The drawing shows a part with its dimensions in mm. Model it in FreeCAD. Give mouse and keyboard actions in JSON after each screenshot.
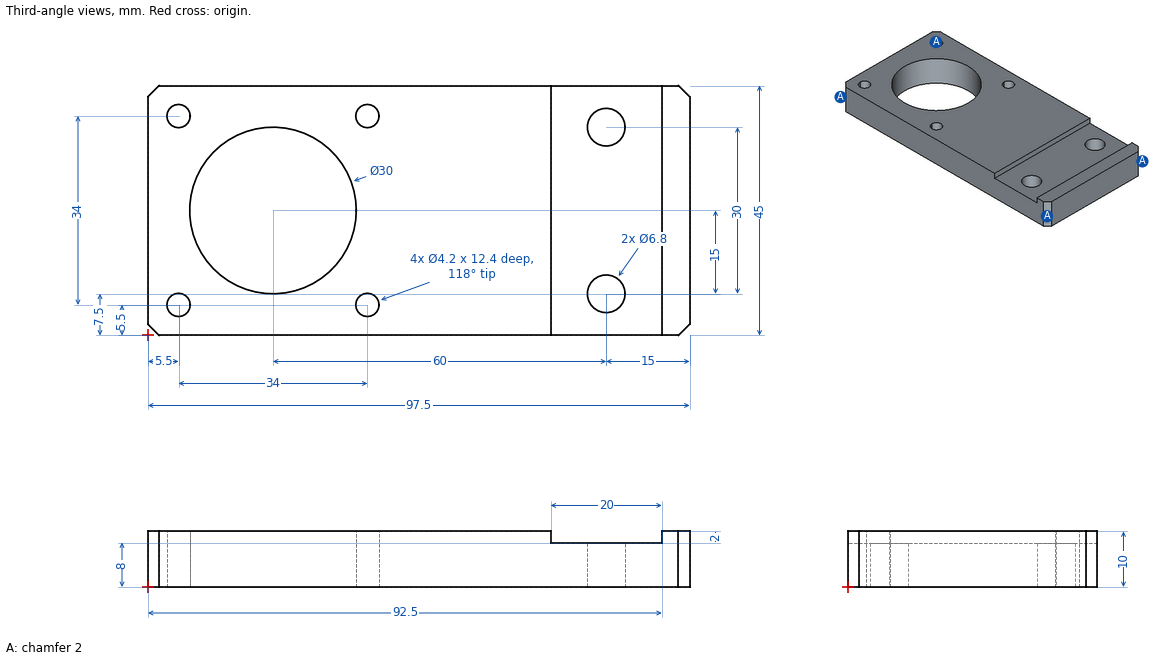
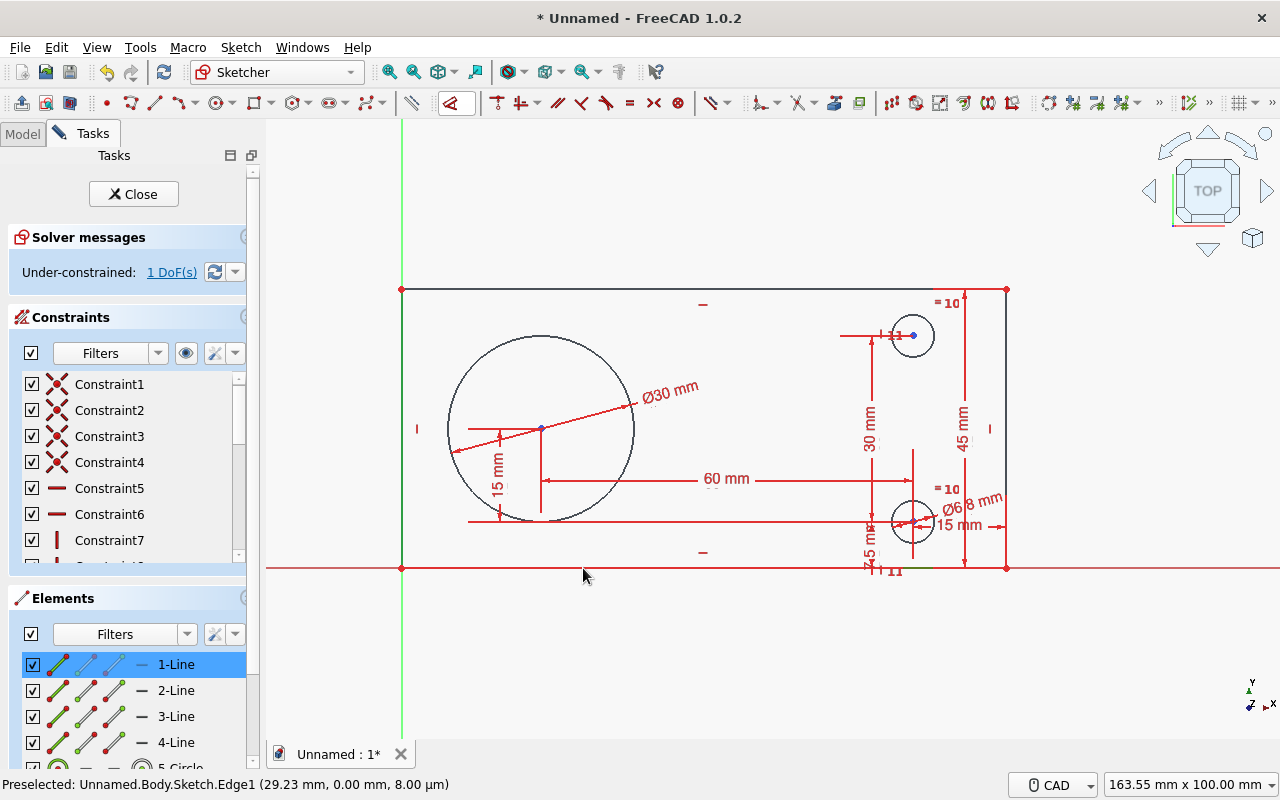
{"action": "key", "text": "l"}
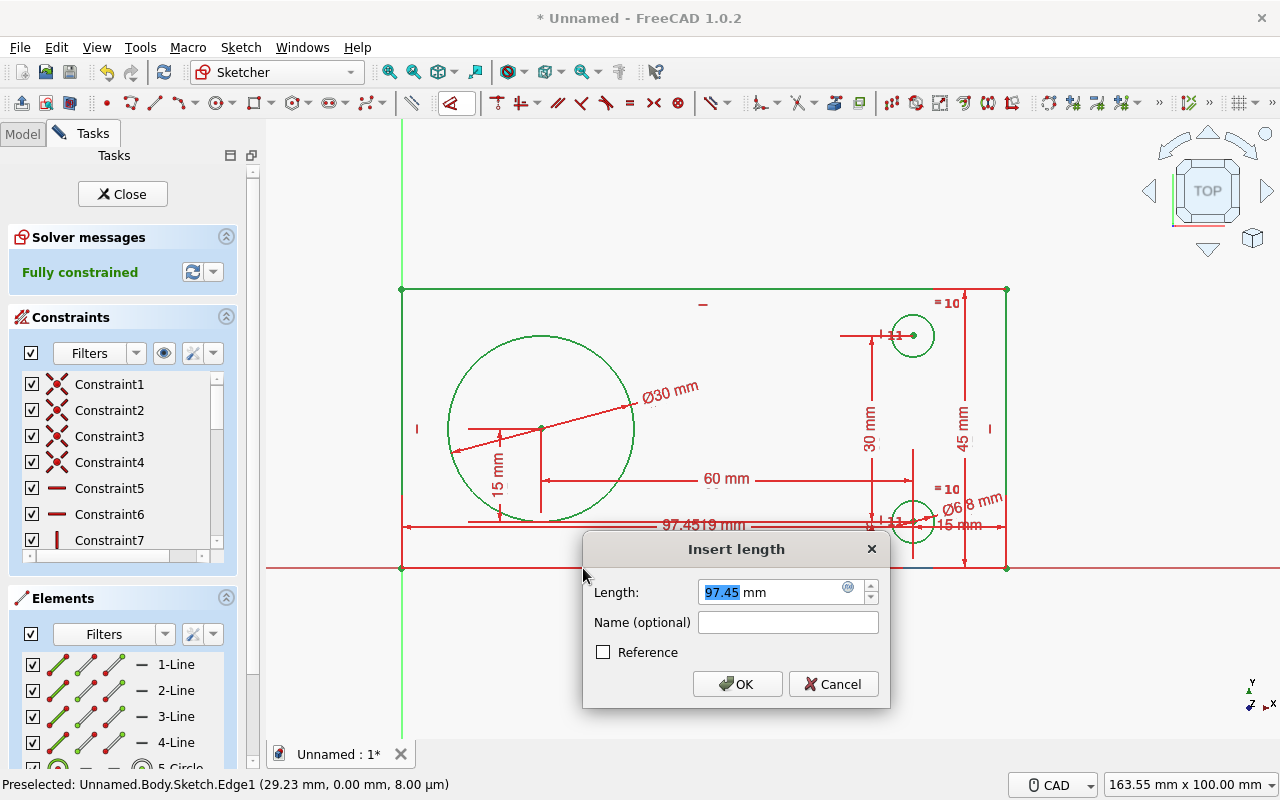
{"action": "type", "text": "97.5"}
{"action": "key", "text": "Return"}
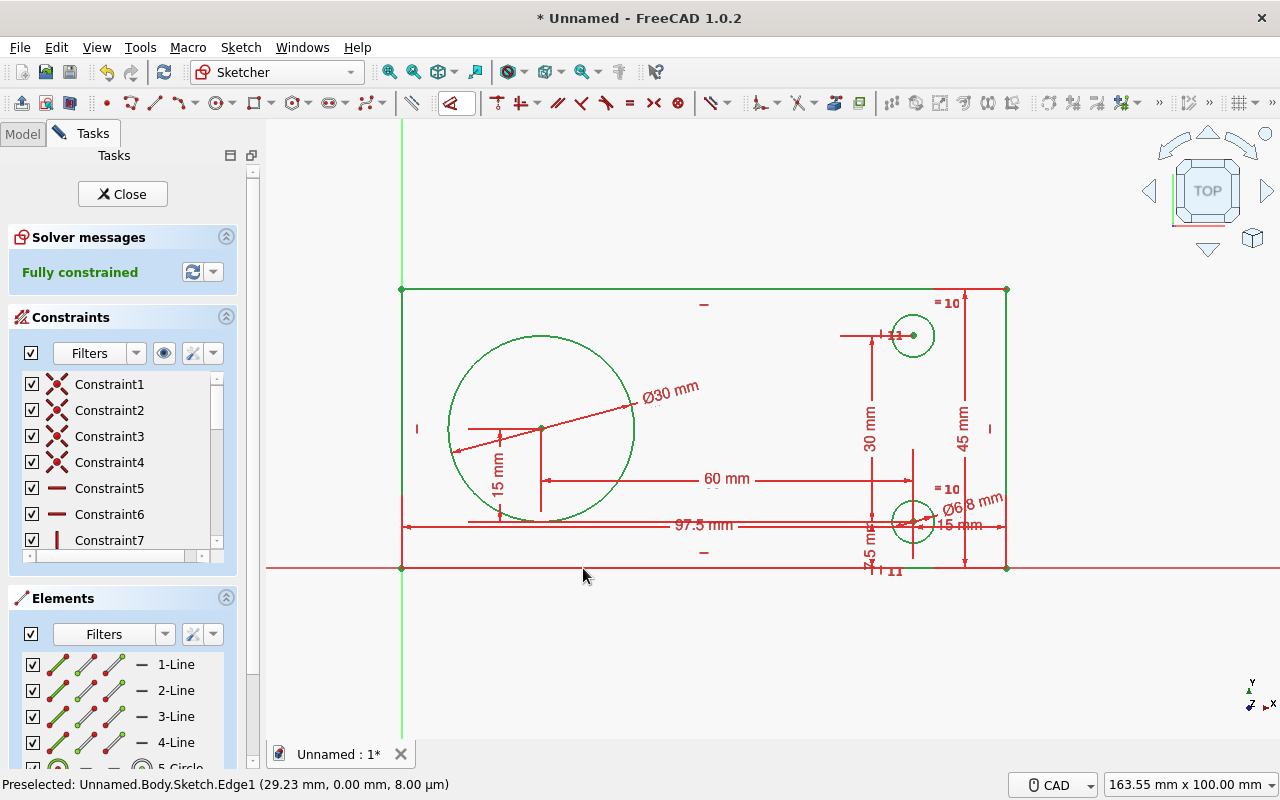
{"action": "left_click", "coordinate": [123, 194]}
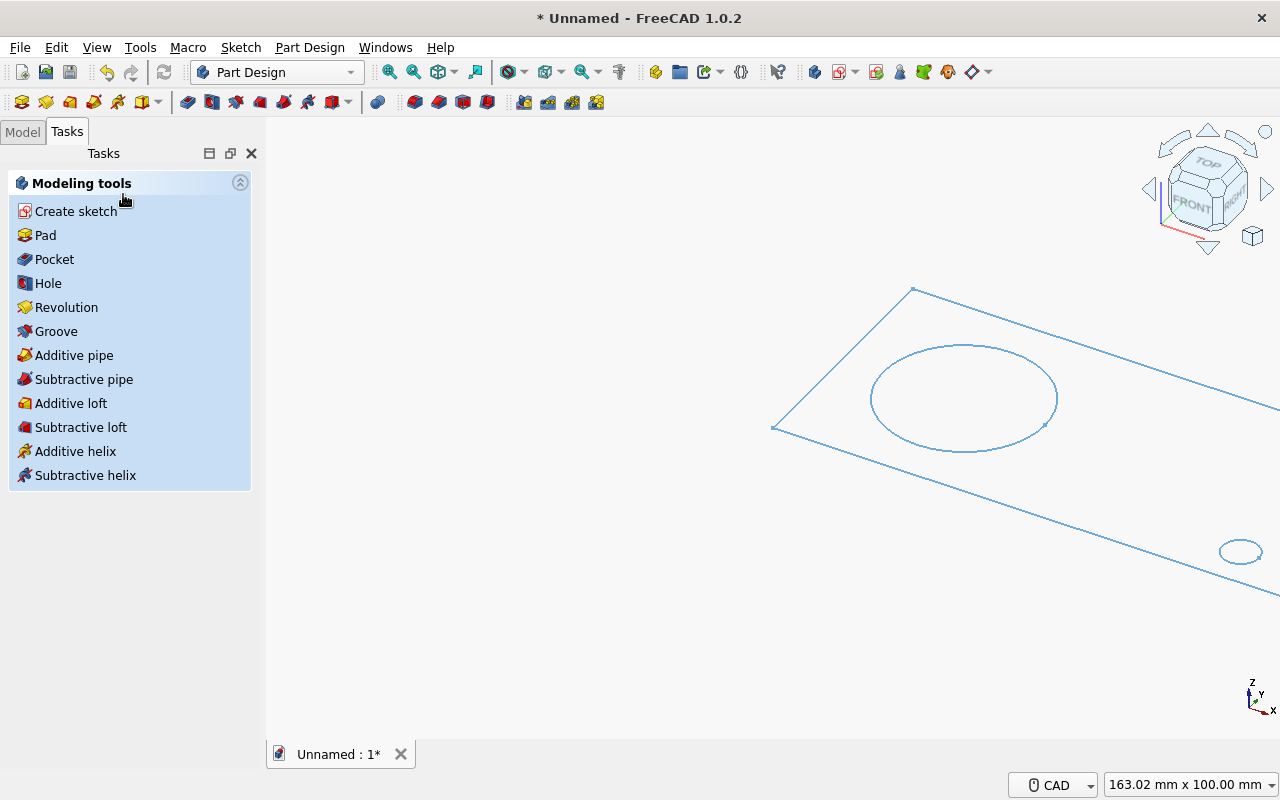
{"action": "left_click", "coordinate": [22, 102]}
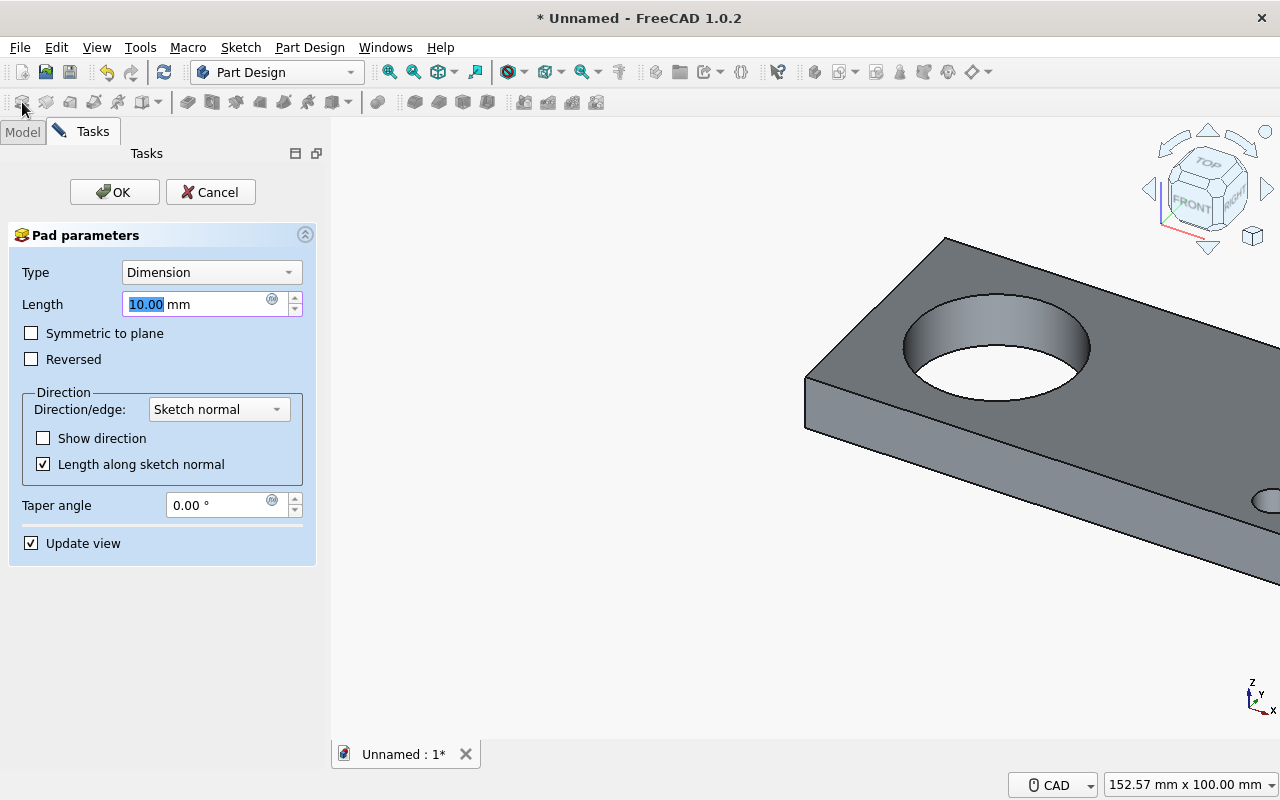
{"action": "type", "text": "10"}
{"action": "key", "text": "Tab"}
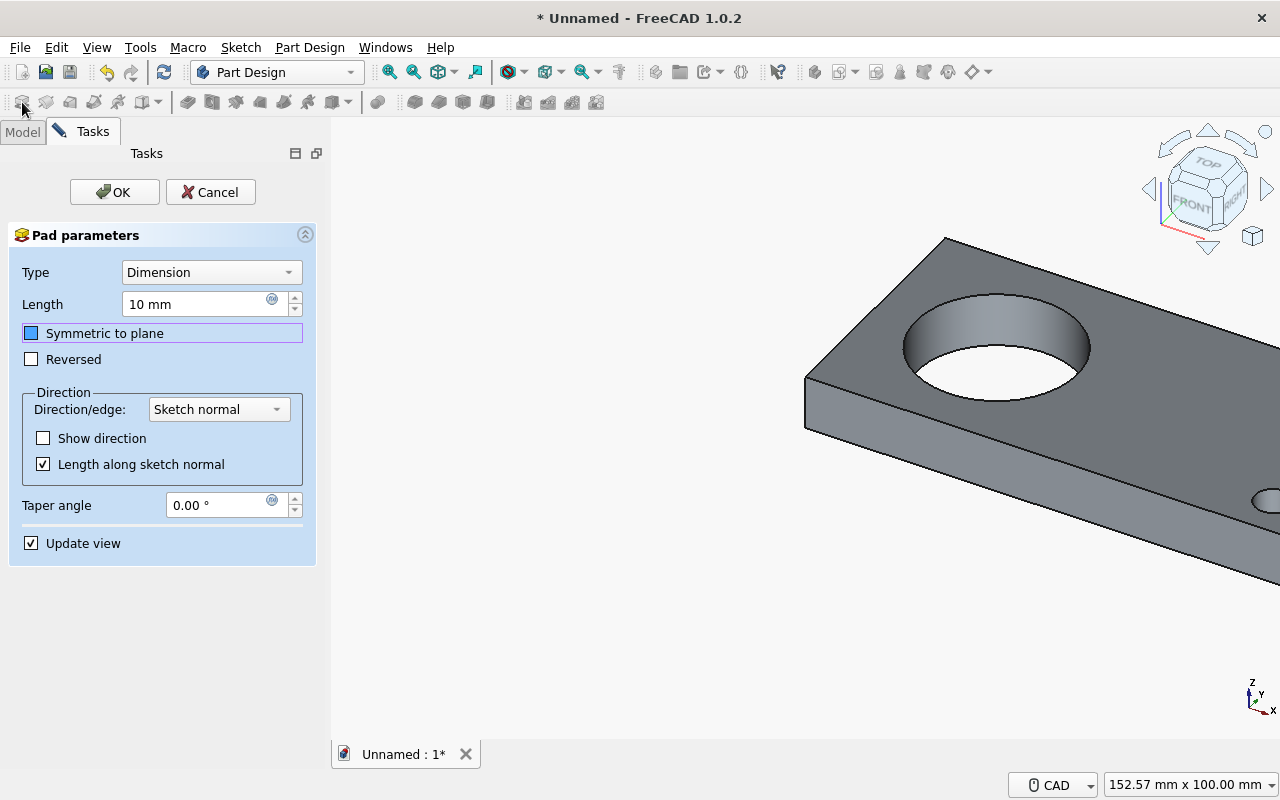
{"action": "left_click", "coordinate": [115, 192]}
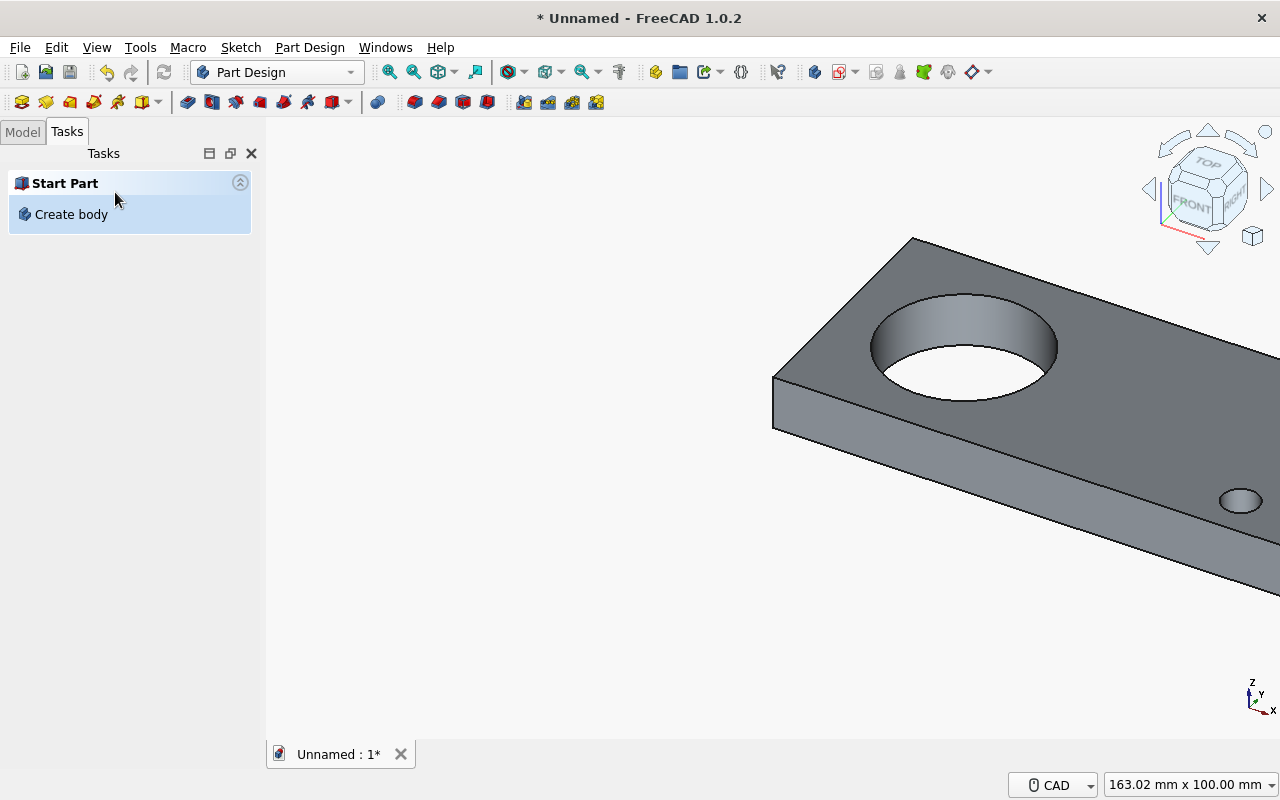
{"action": "left_click", "coordinate": [390, 72]}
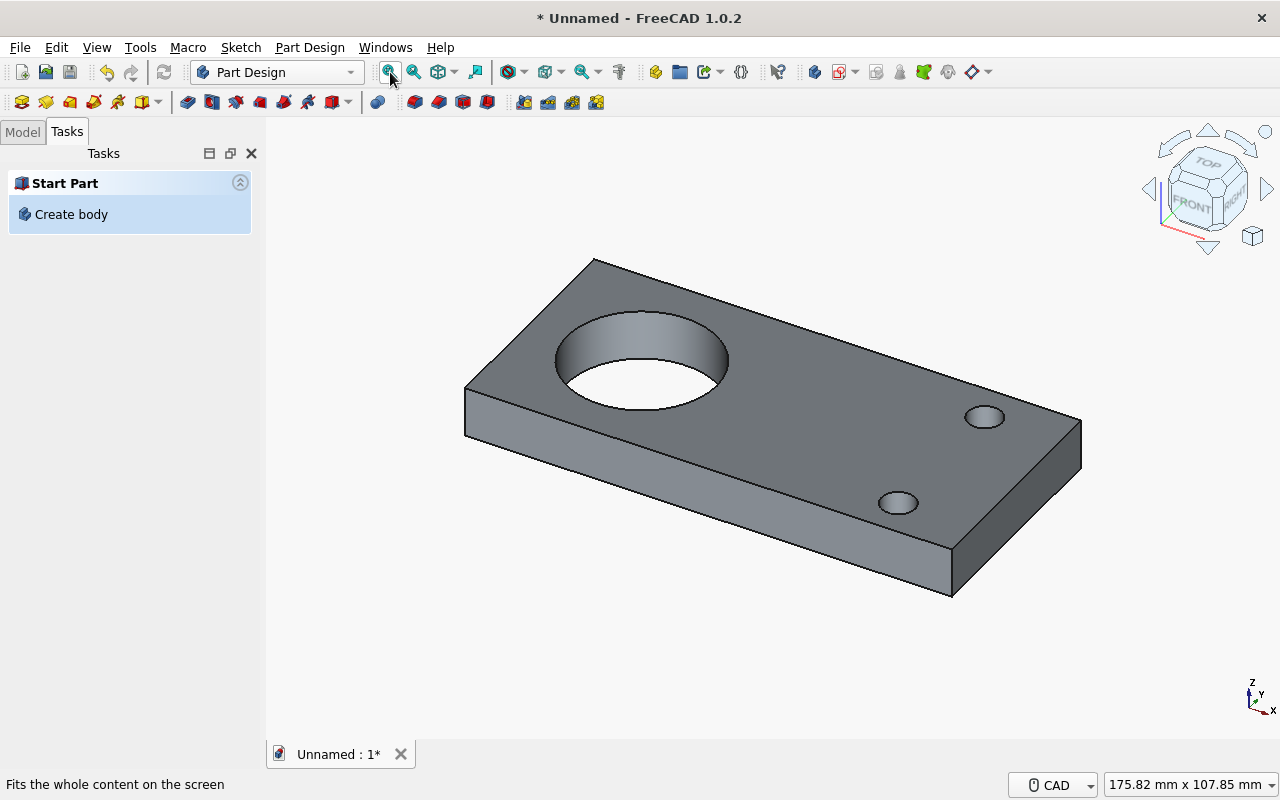
{"action": "key", "text": "4"}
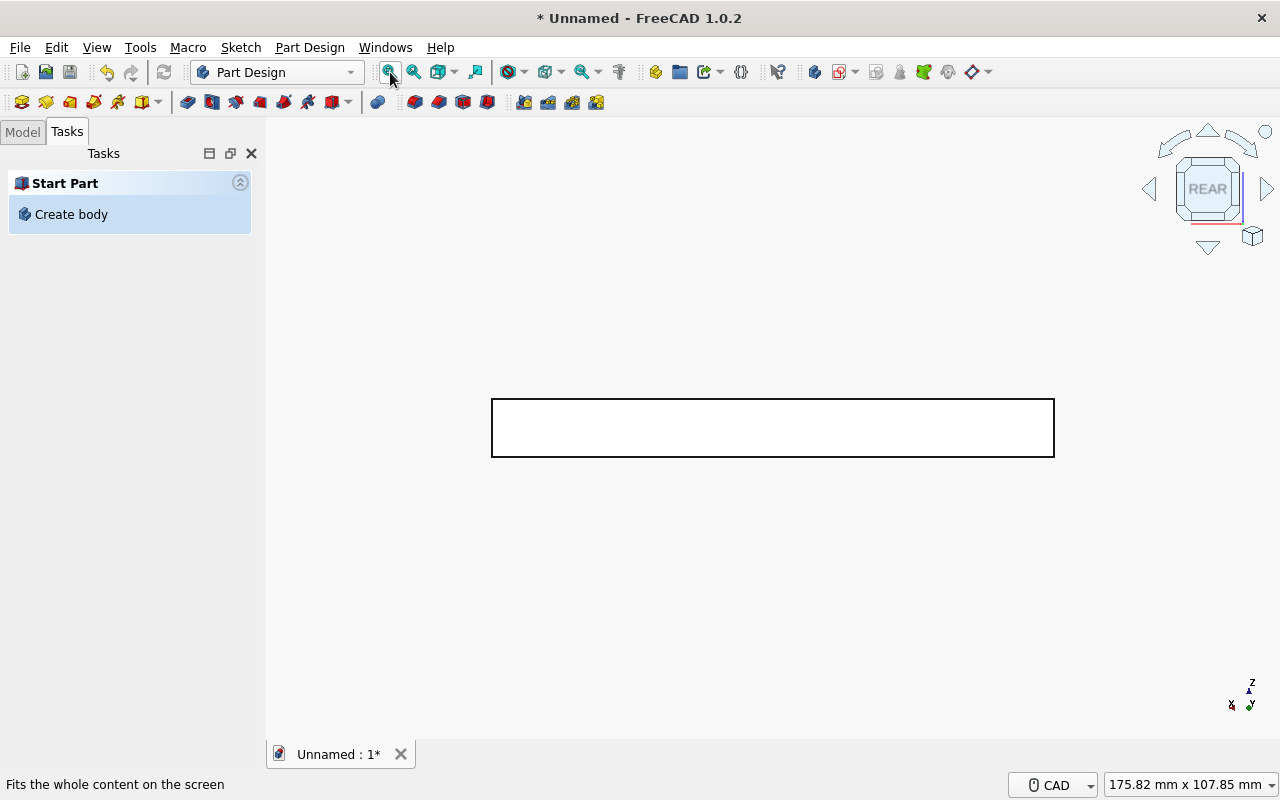
{"action": "left_click", "coordinate": [532, 427]}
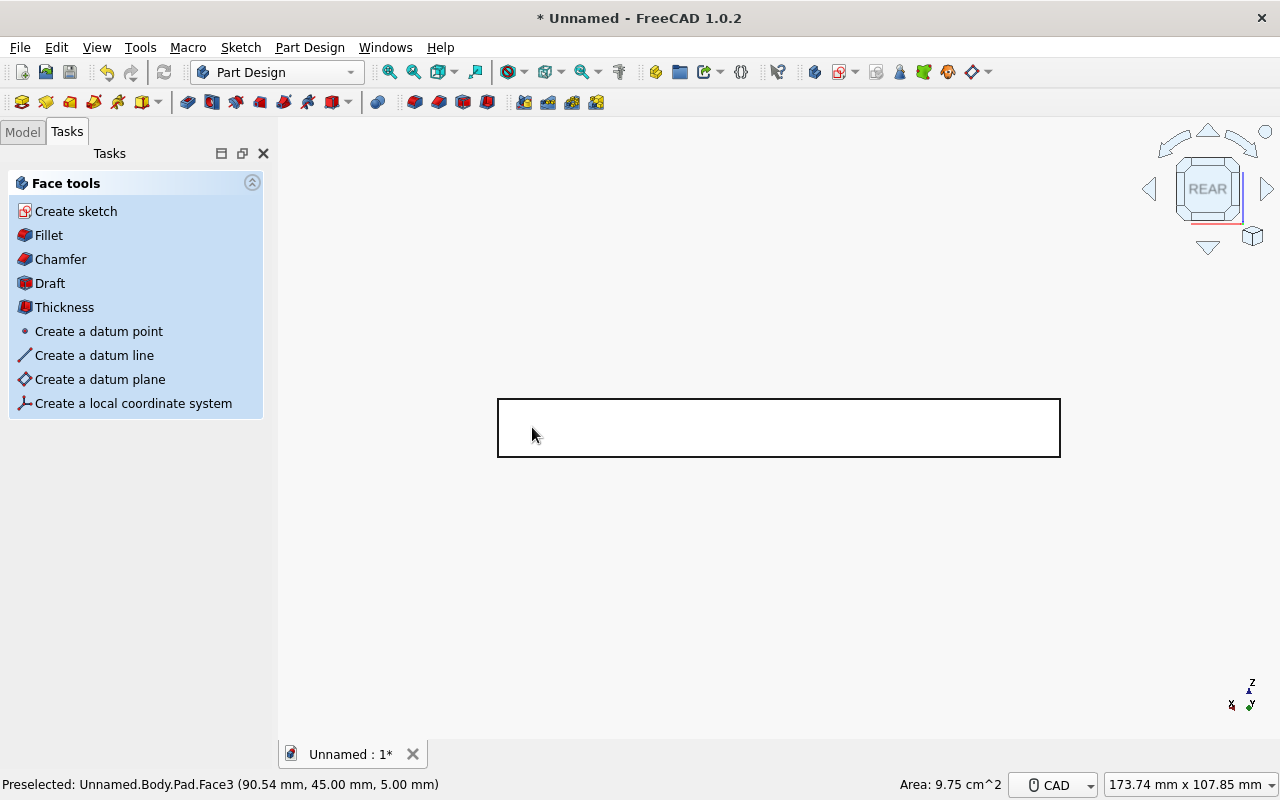
{"action": "left_click", "coordinate": [840, 72]}